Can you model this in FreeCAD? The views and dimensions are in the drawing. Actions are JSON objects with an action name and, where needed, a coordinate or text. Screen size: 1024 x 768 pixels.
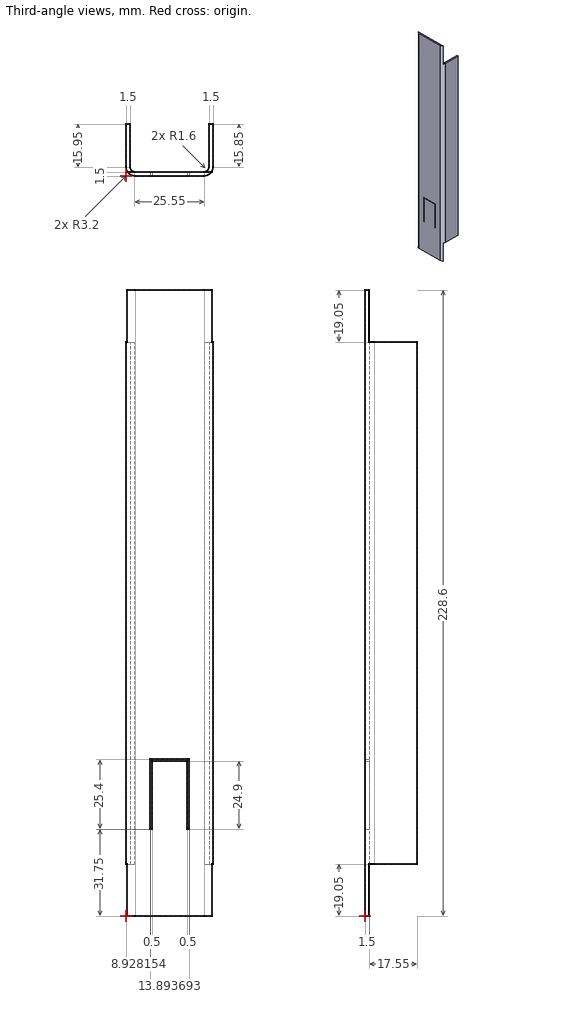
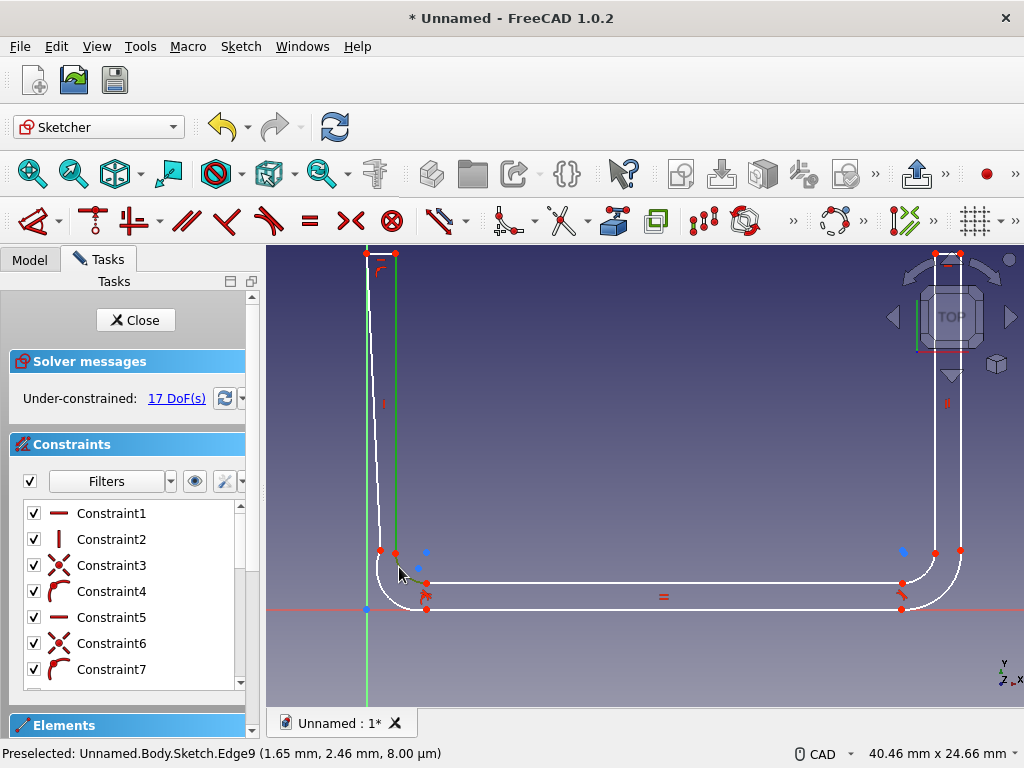
{"action": "left_click", "coordinate": [269, 222]}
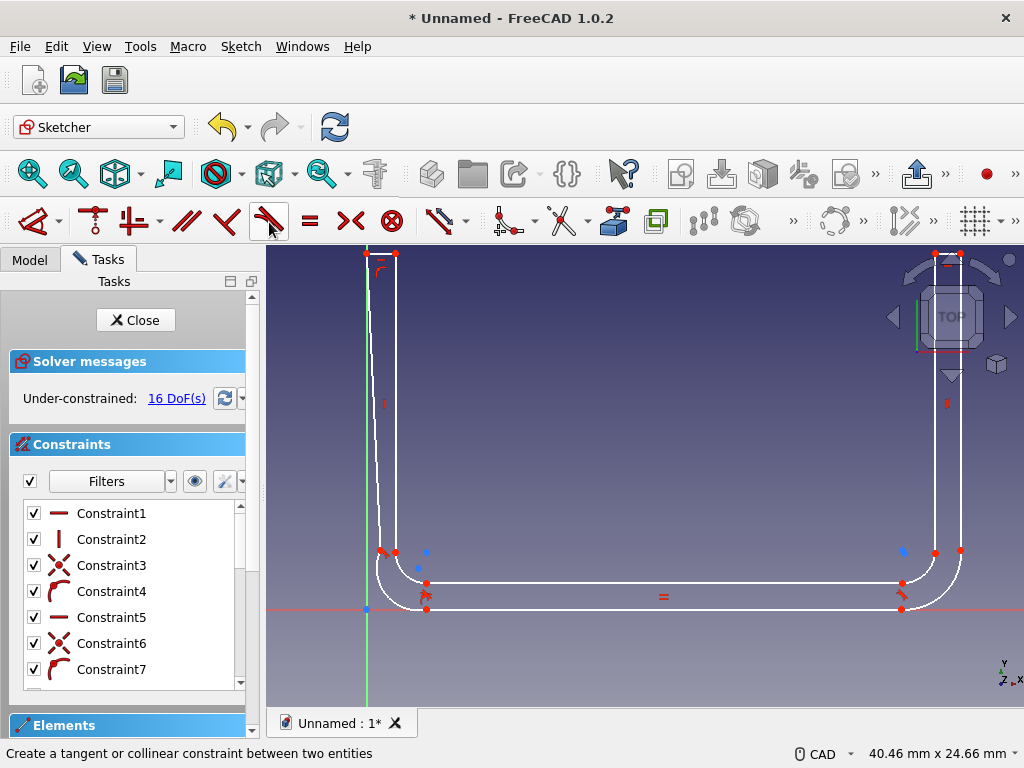
{"action": "scroll", "coordinate": [376, 461], "scroll_direction": "up", "scroll_amount": 2}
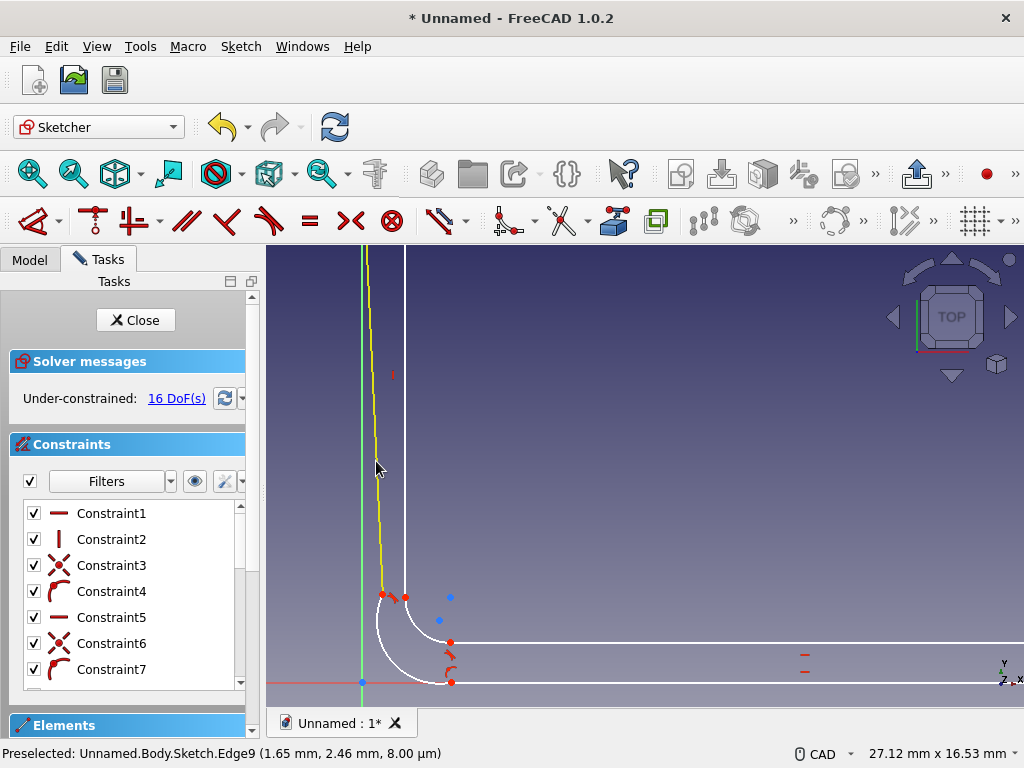
{"action": "left_click", "coordinate": [377, 461]}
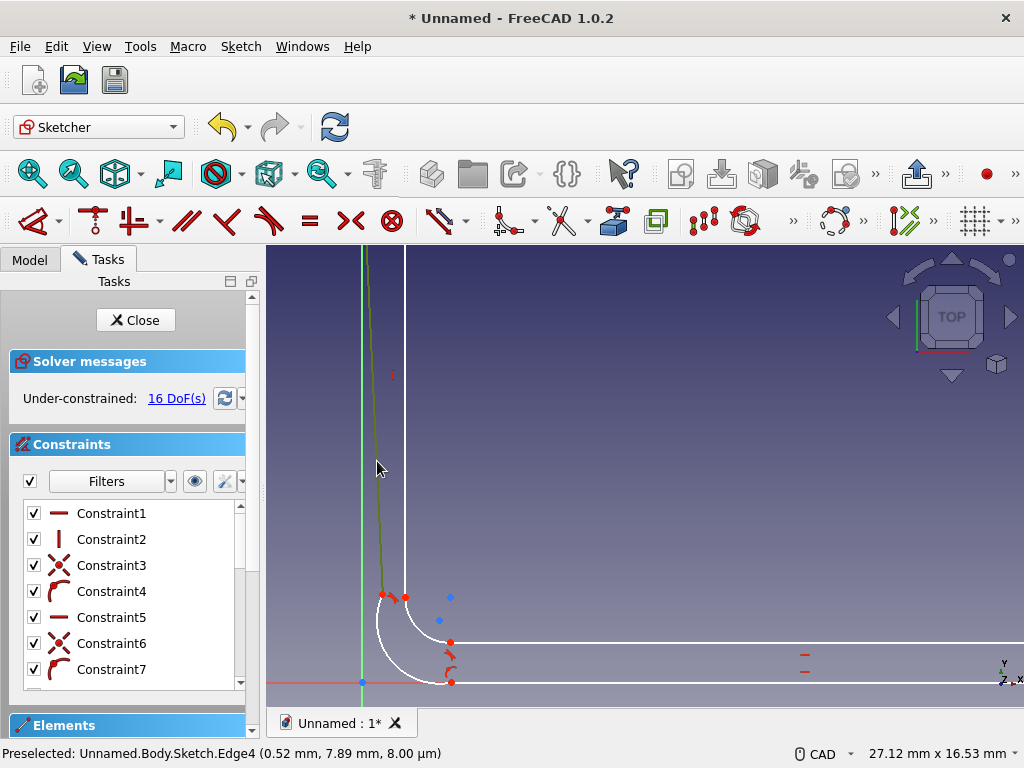
{"action": "left_click", "coordinate": [379, 635]}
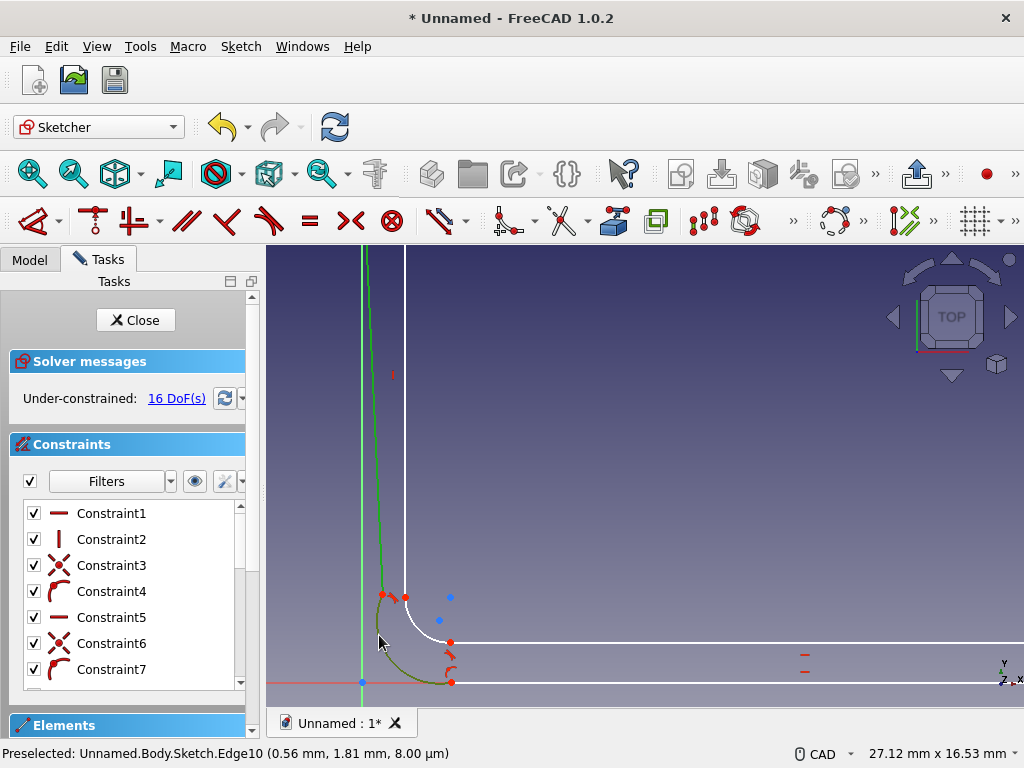
{"action": "left_click", "coordinate": [269, 222]}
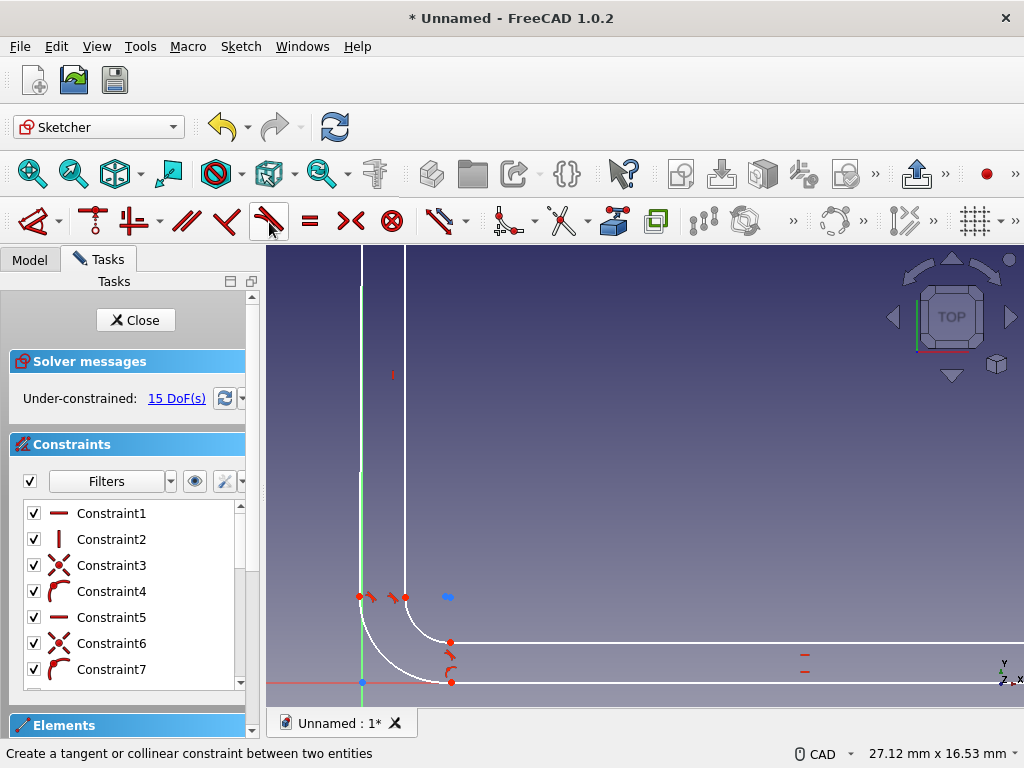
{"action": "scroll", "coordinate": [389, 525], "scroll_direction": "down", "scroll_amount": 4}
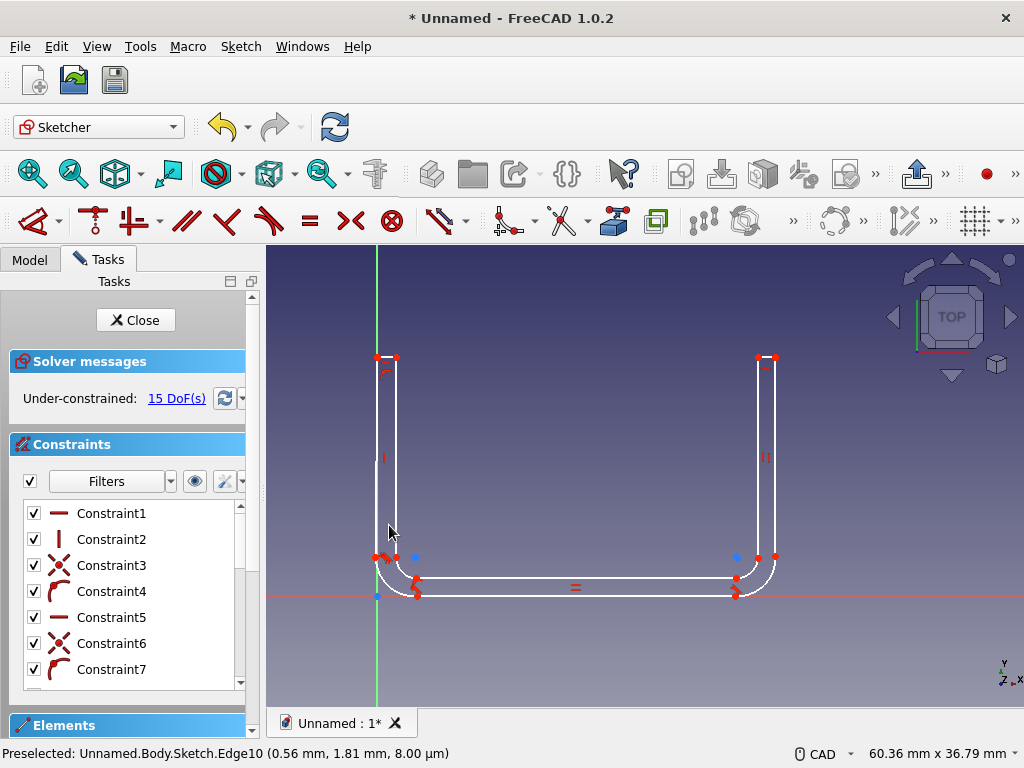
{"action": "left_click", "coordinate": [513, 596]}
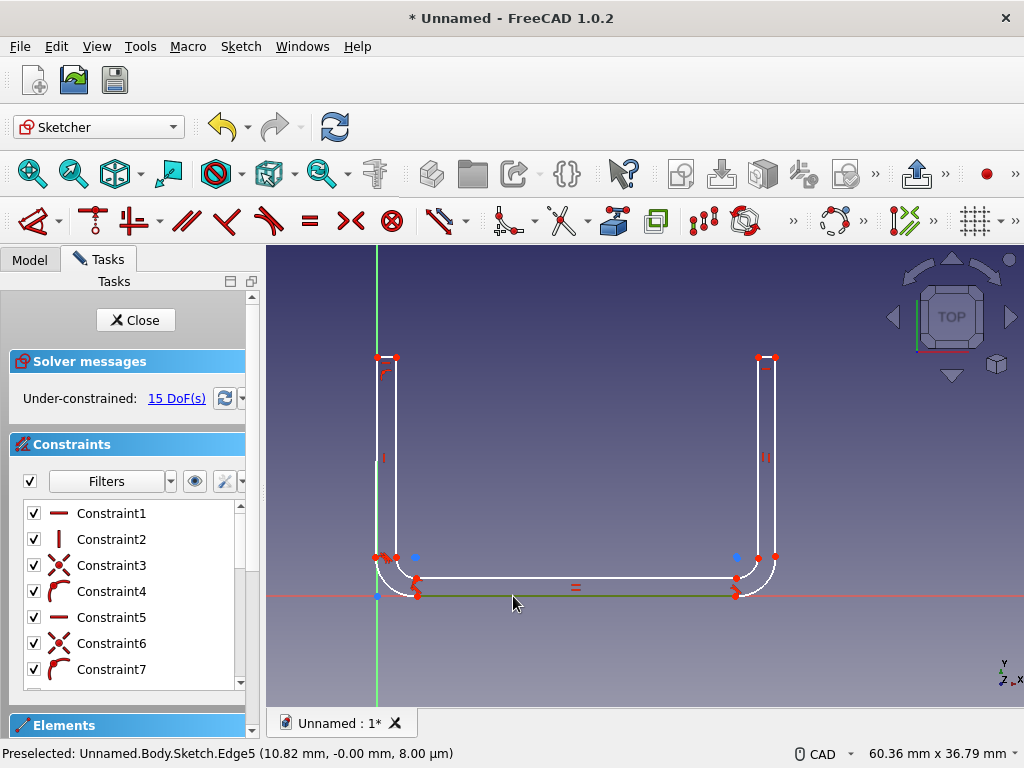
{"action": "left_click", "coordinate": [381, 576]}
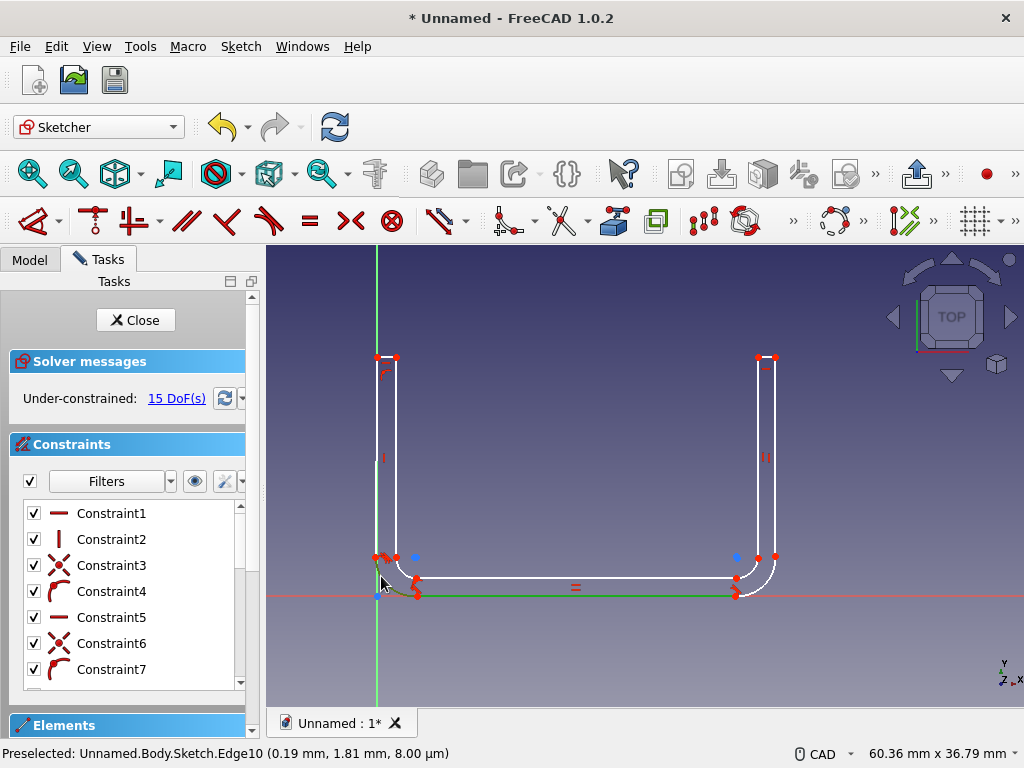
{"action": "left_click", "coordinate": [269, 222]}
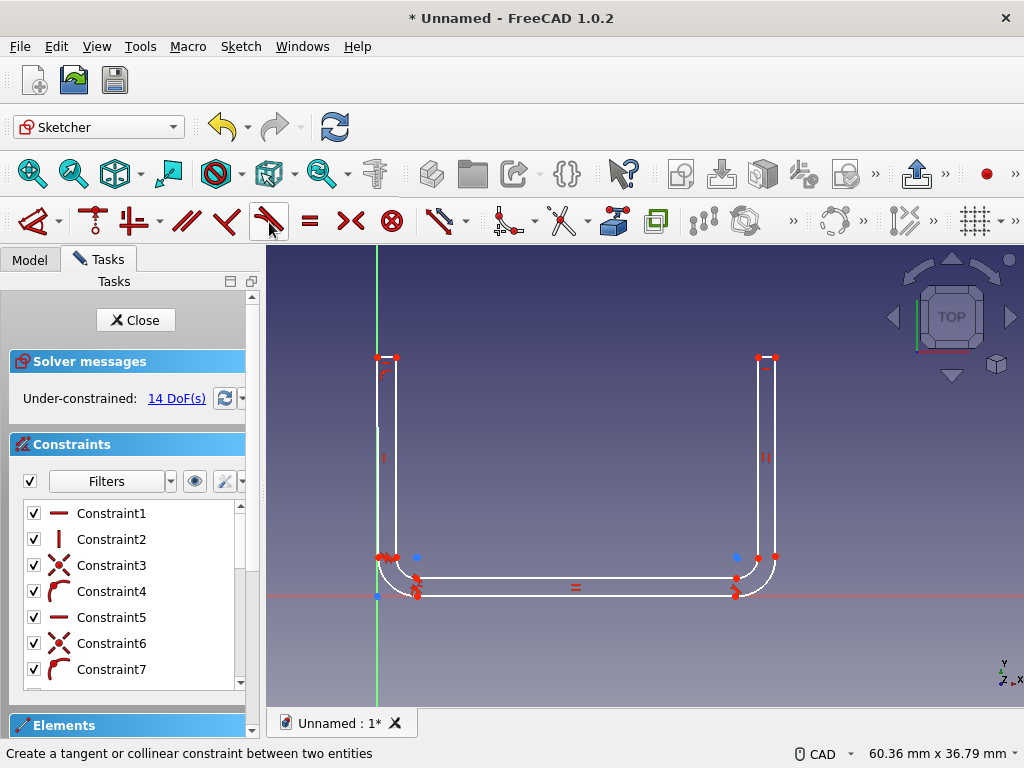
{"action": "left_click", "coordinate": [513, 596]}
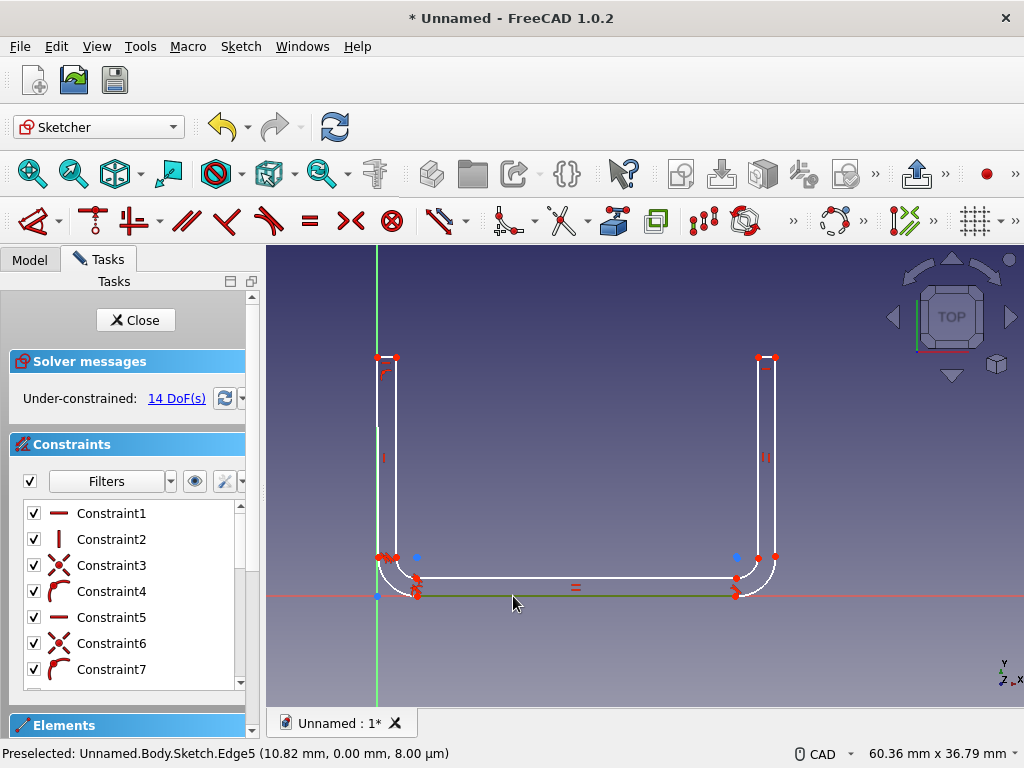
{"action": "left_click", "coordinate": [754, 592]}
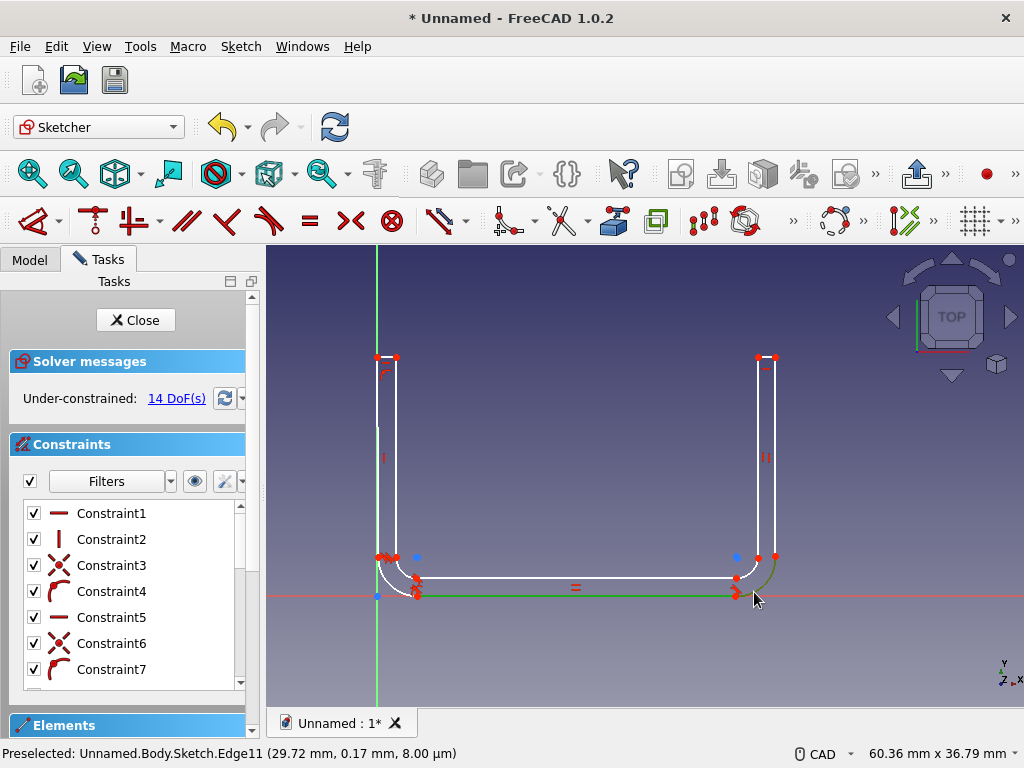
{"action": "left_click", "coordinate": [269, 222]}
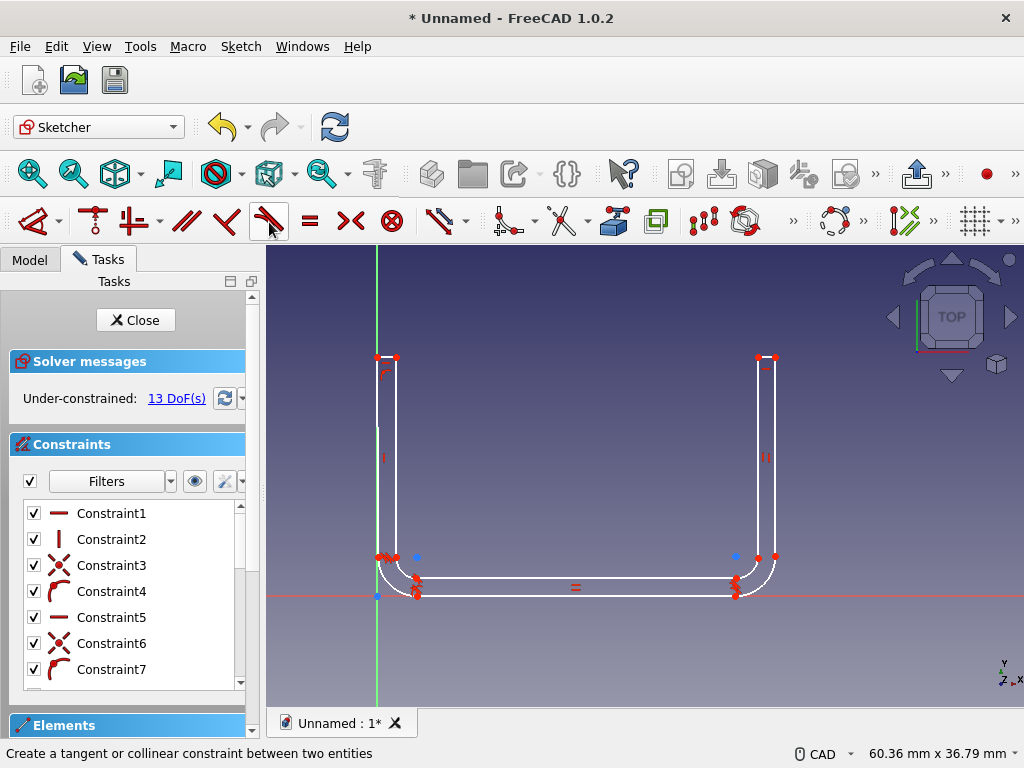
{"action": "left_click", "coordinate": [775, 497]}